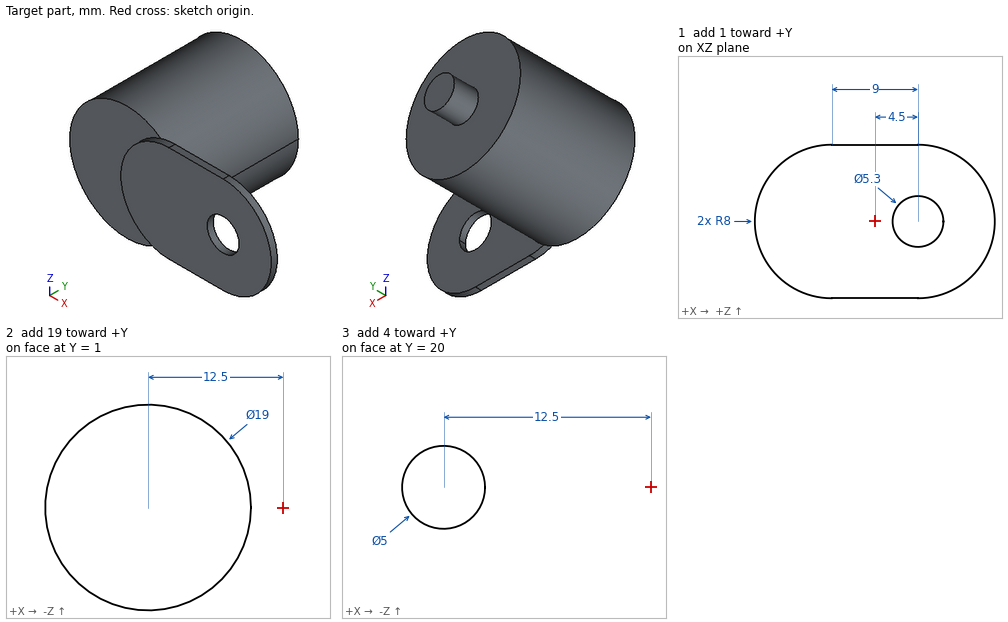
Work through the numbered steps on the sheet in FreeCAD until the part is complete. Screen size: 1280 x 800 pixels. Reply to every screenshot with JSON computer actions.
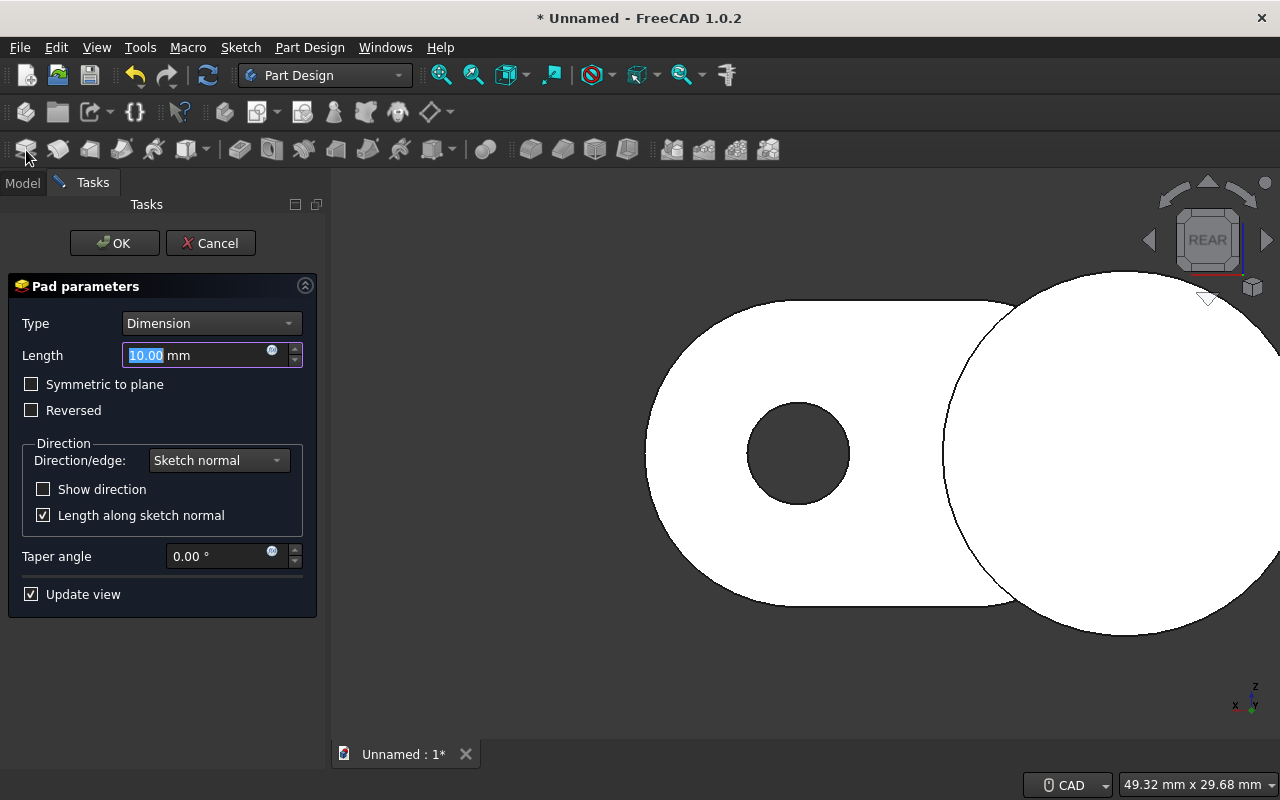
{"action": "type", "text": "19"}
{"action": "key", "text": "Tab"}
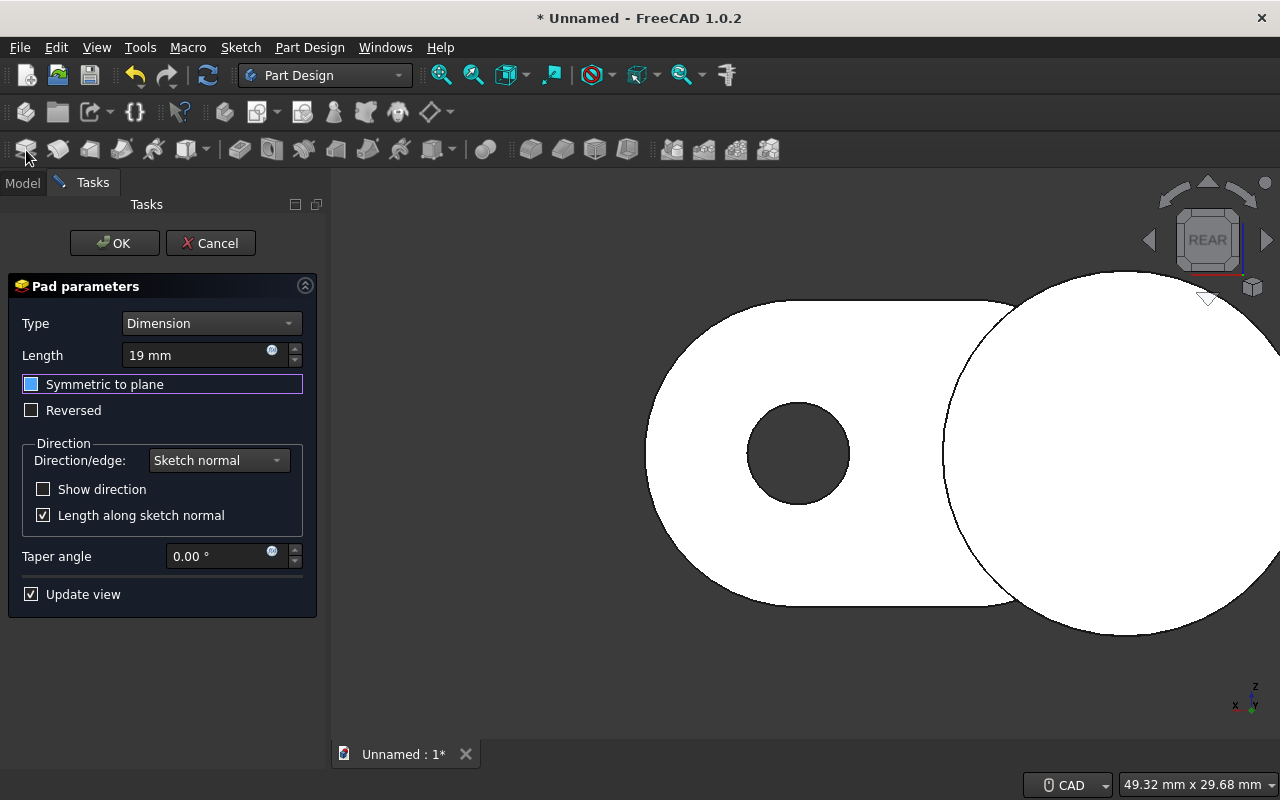
{"action": "left_click", "coordinate": [115, 243]}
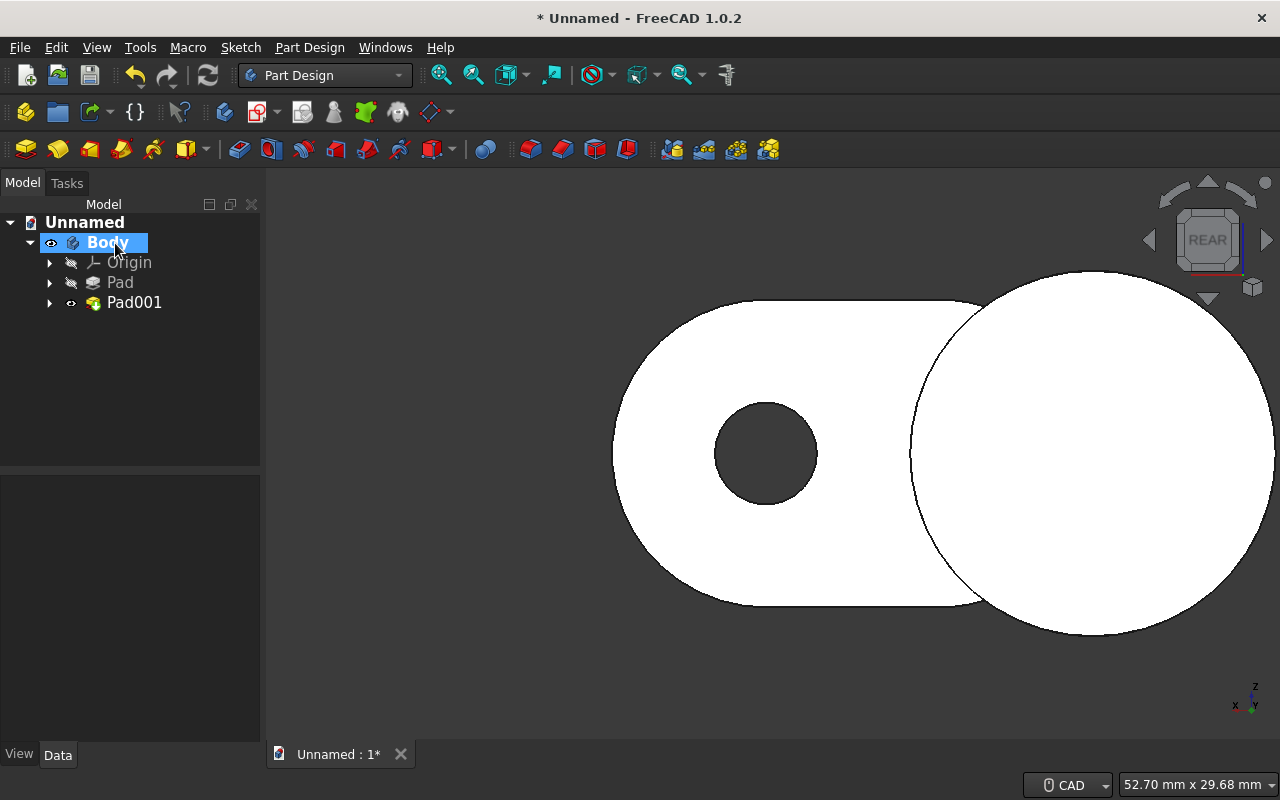
{"action": "left_click", "coordinate": [1093, 453]}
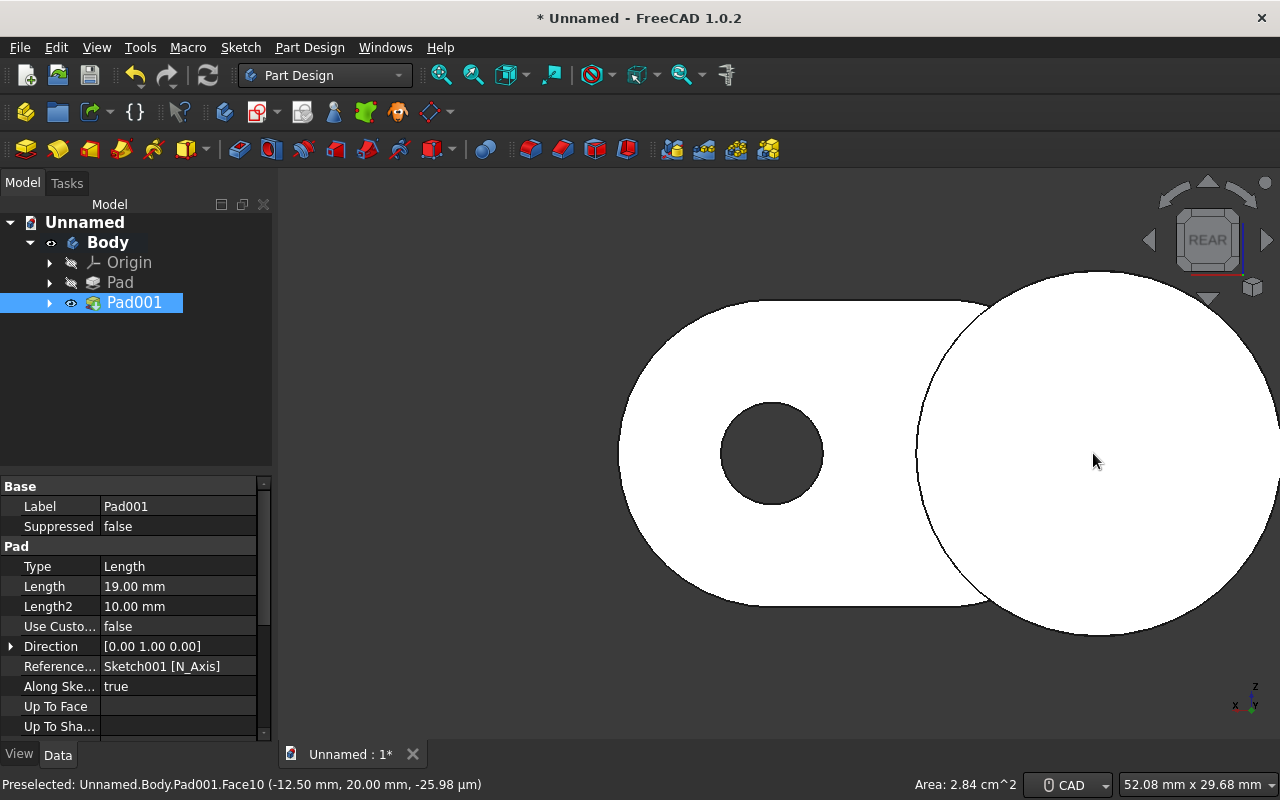
{"action": "left_click", "coordinate": [258, 112]}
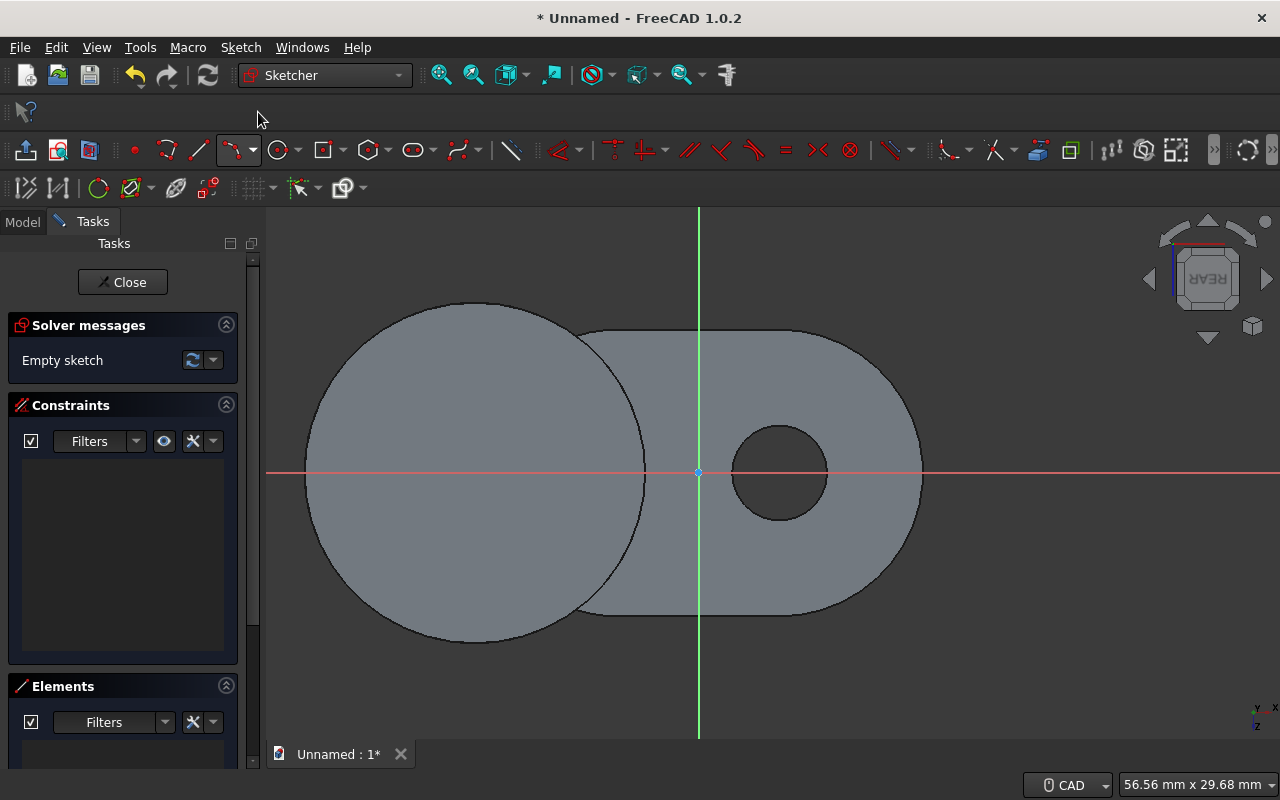
{"action": "scroll", "coordinate": [400, 473], "scroll_direction": "up", "scroll_amount": 7}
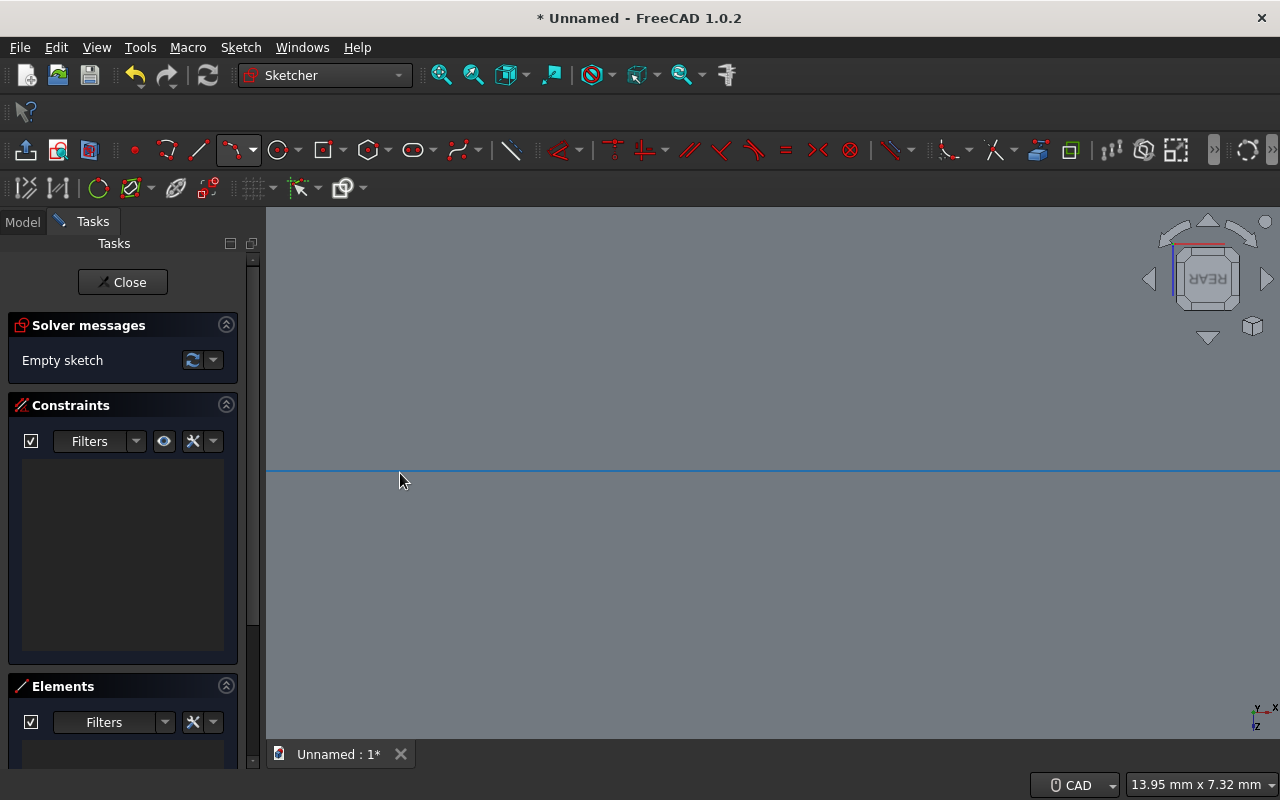
{"action": "left_click", "coordinate": [278, 150]}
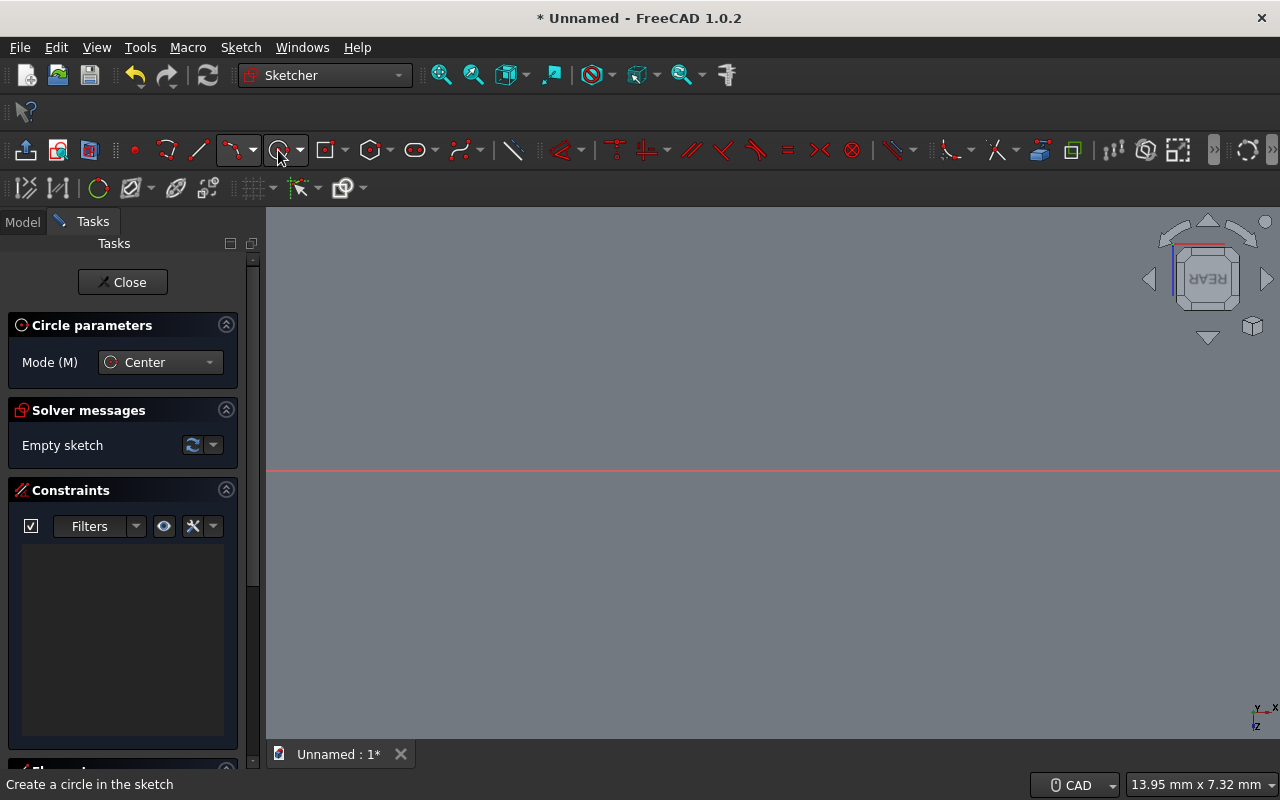
{"action": "left_click", "coordinate": [703, 471]}
{"action": "left_click", "coordinate": [832, 343]}
{"action": "key", "text": "Escape"}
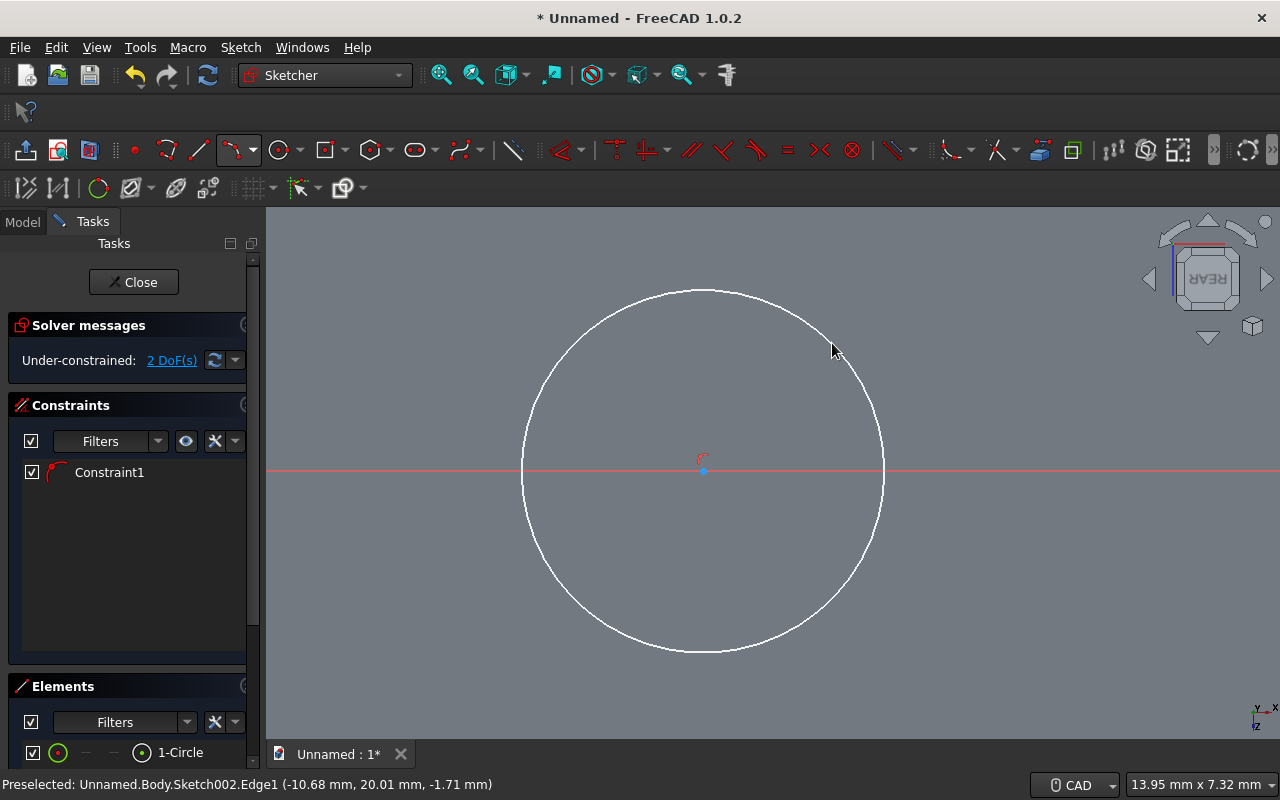
{"action": "left_click", "coordinate": [560, 150]}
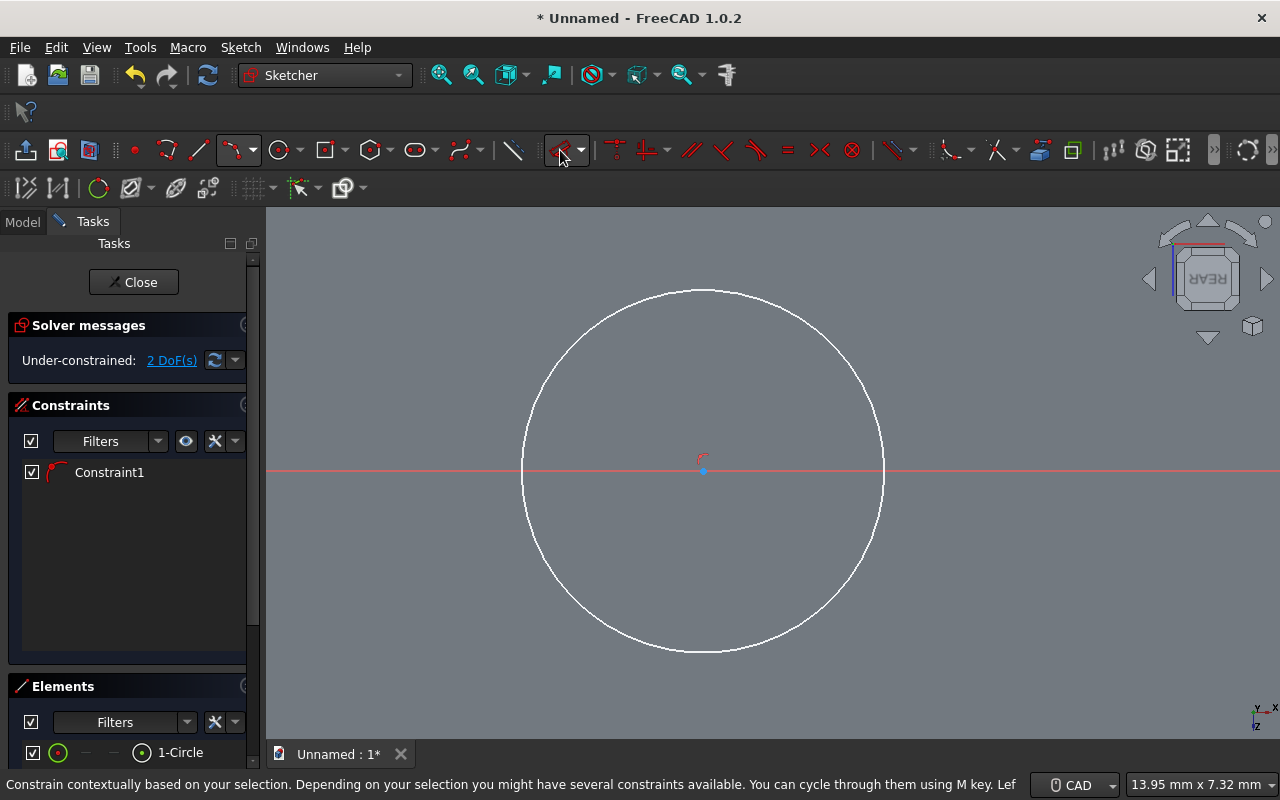
{"action": "left_click", "coordinate": [831, 343]}
{"action": "left_click", "coordinate": [854, 320]}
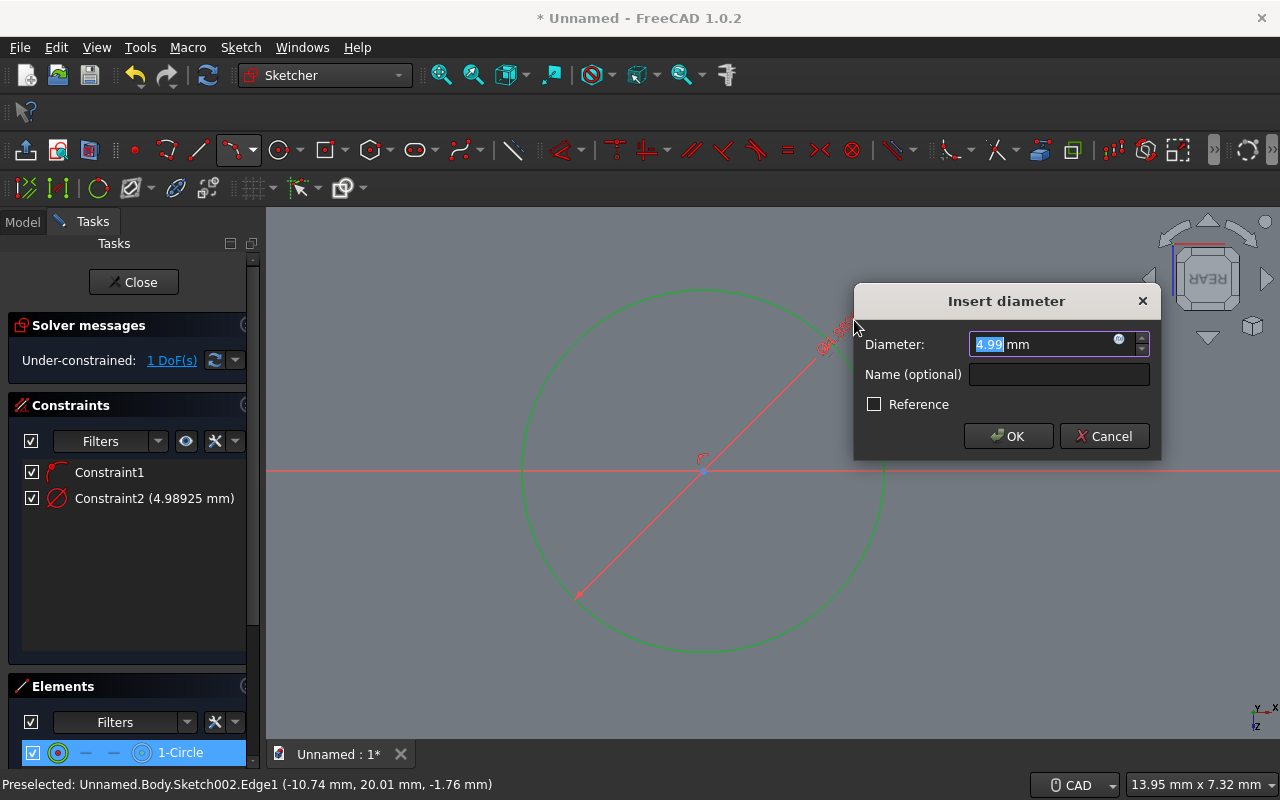
{"action": "type", "text": "5"}
{"action": "key", "text": "Return"}